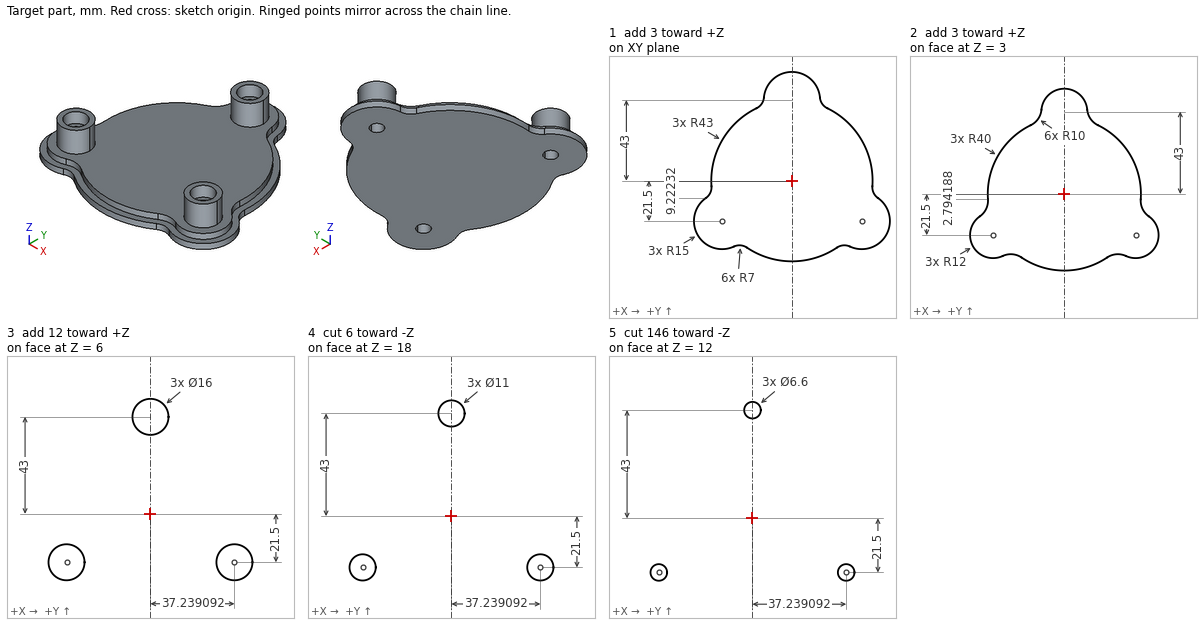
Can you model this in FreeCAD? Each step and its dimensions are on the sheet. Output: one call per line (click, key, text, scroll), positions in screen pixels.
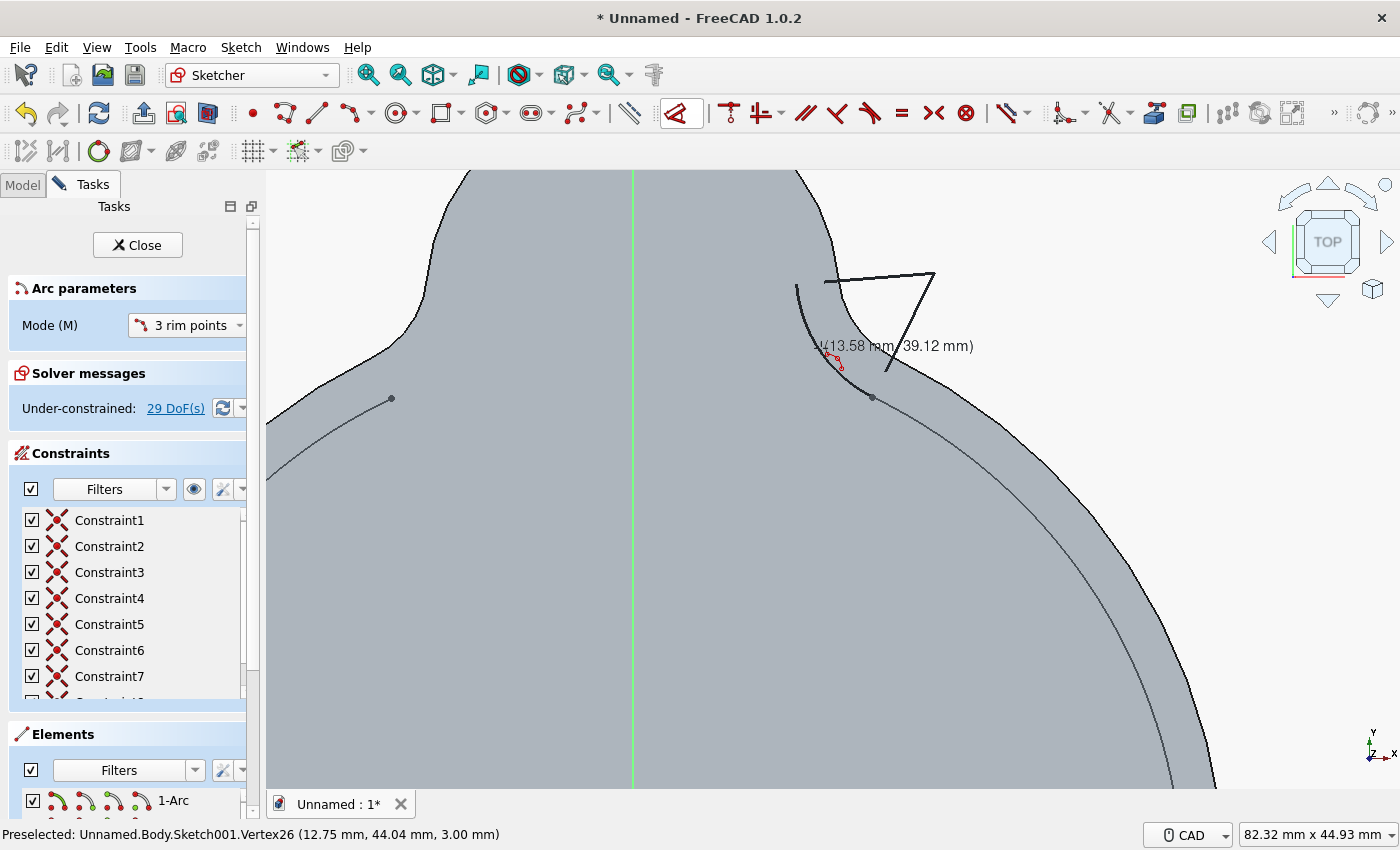
click(821, 349)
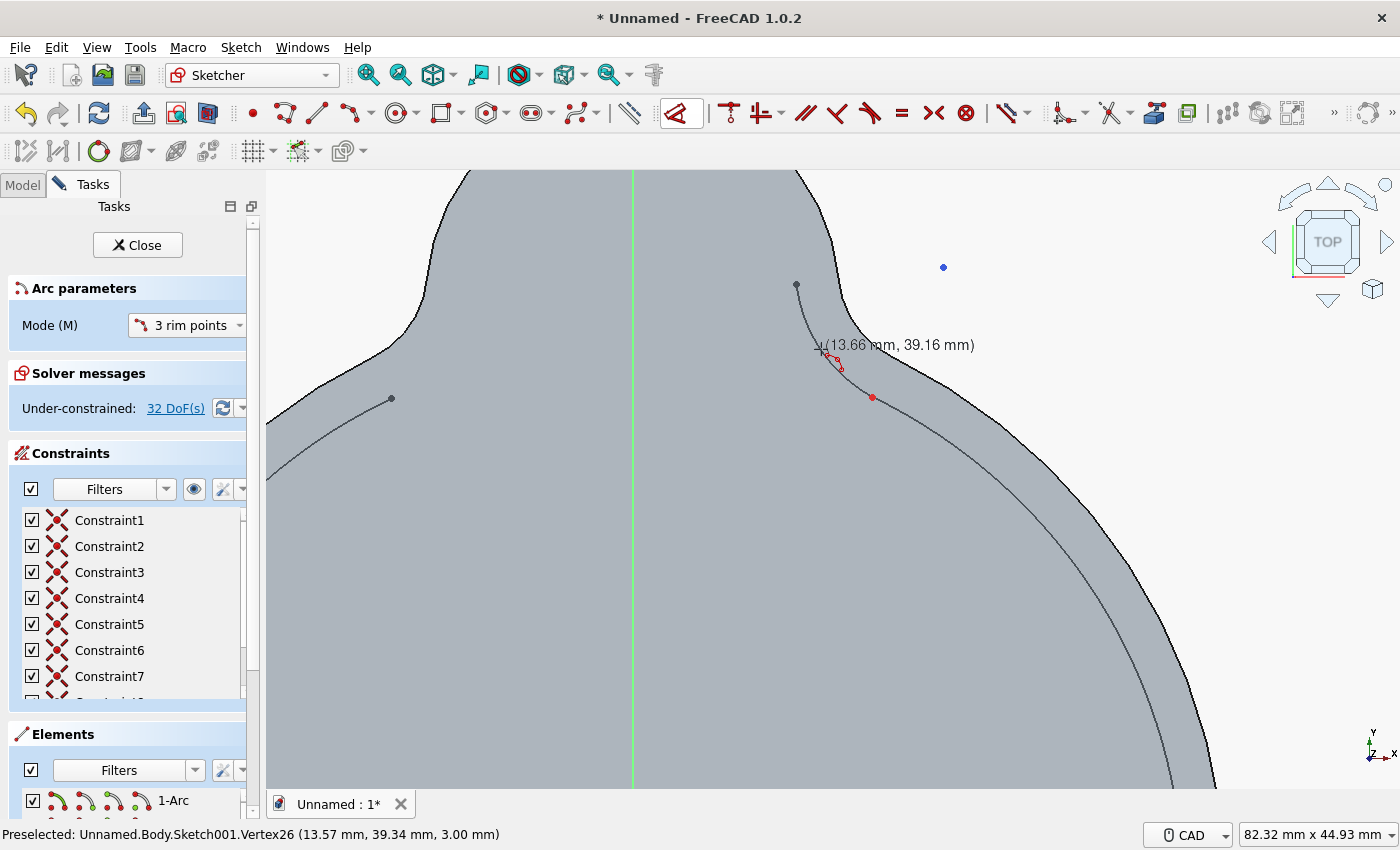
click(797, 284)
click(468, 283)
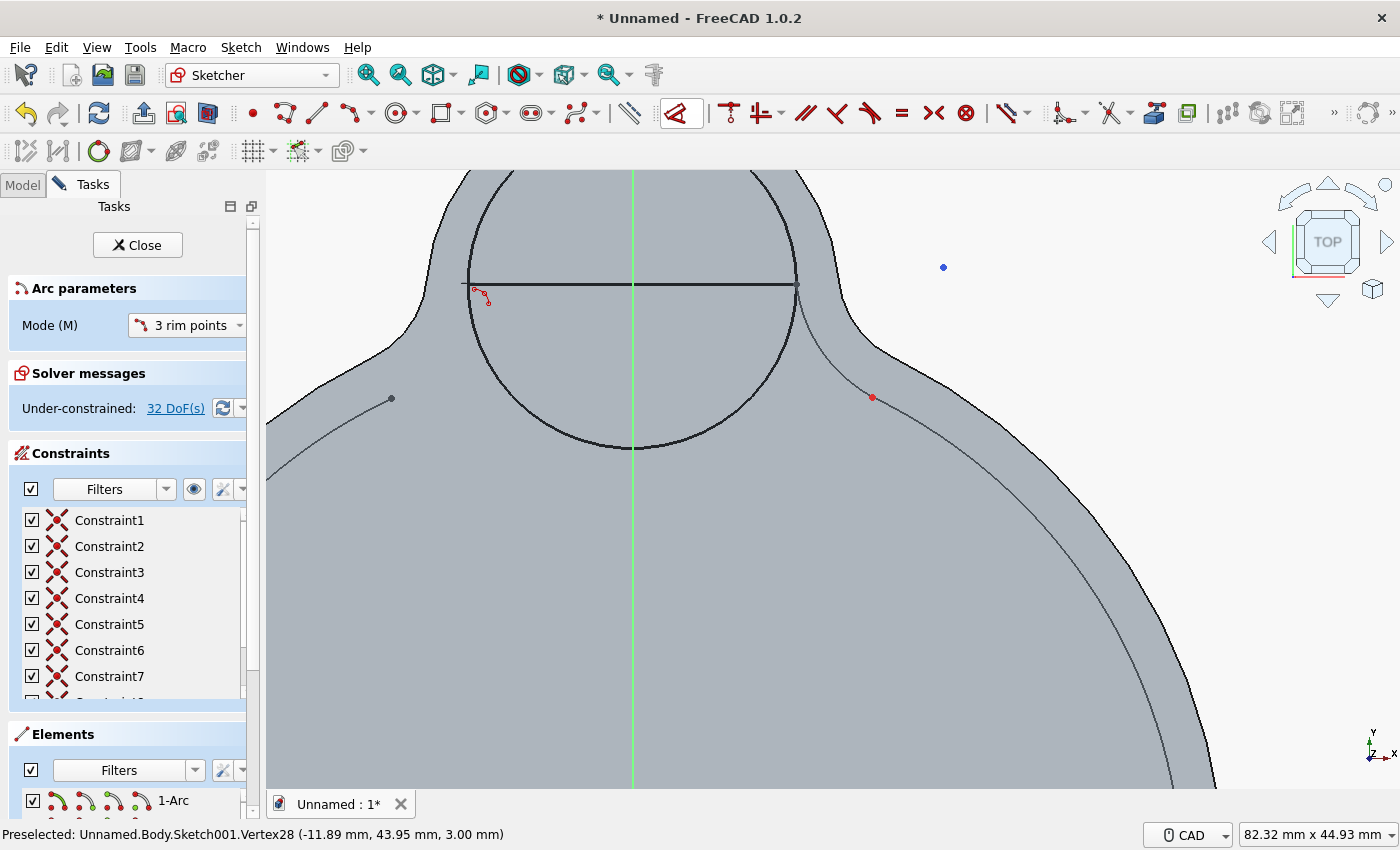
scroll(821, 347, down, 6)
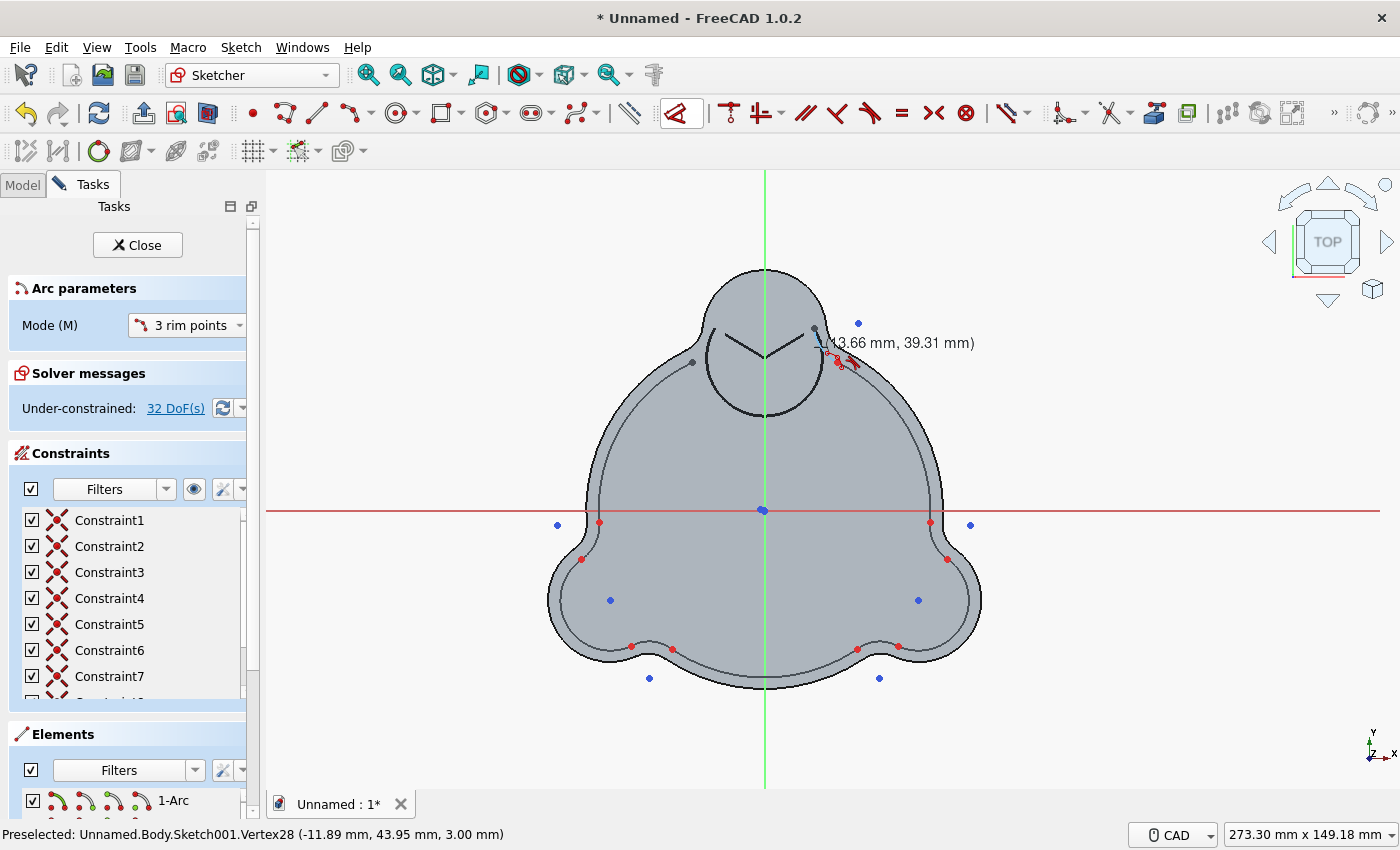
click(779, 285)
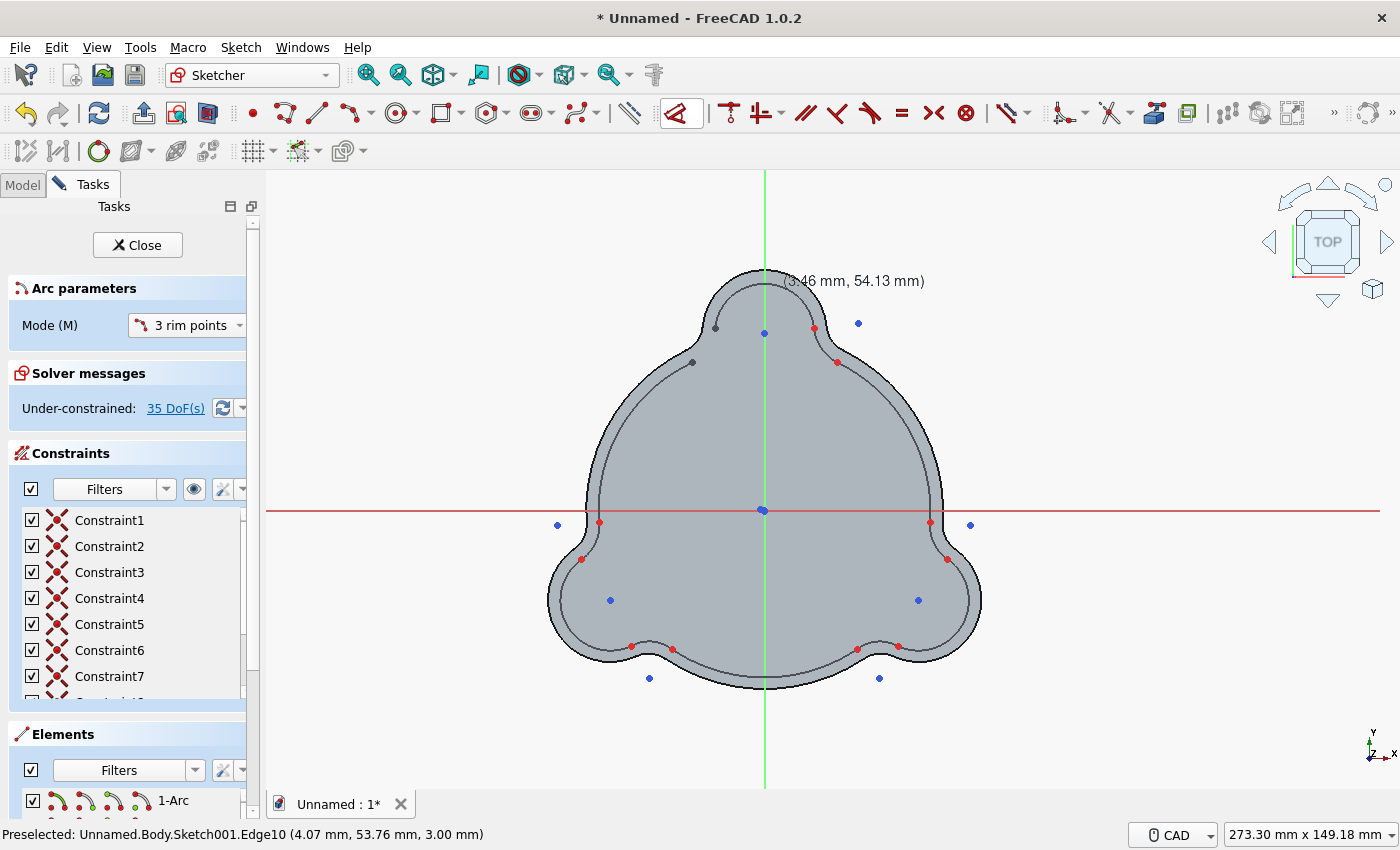
click(715, 328)
click(692, 363)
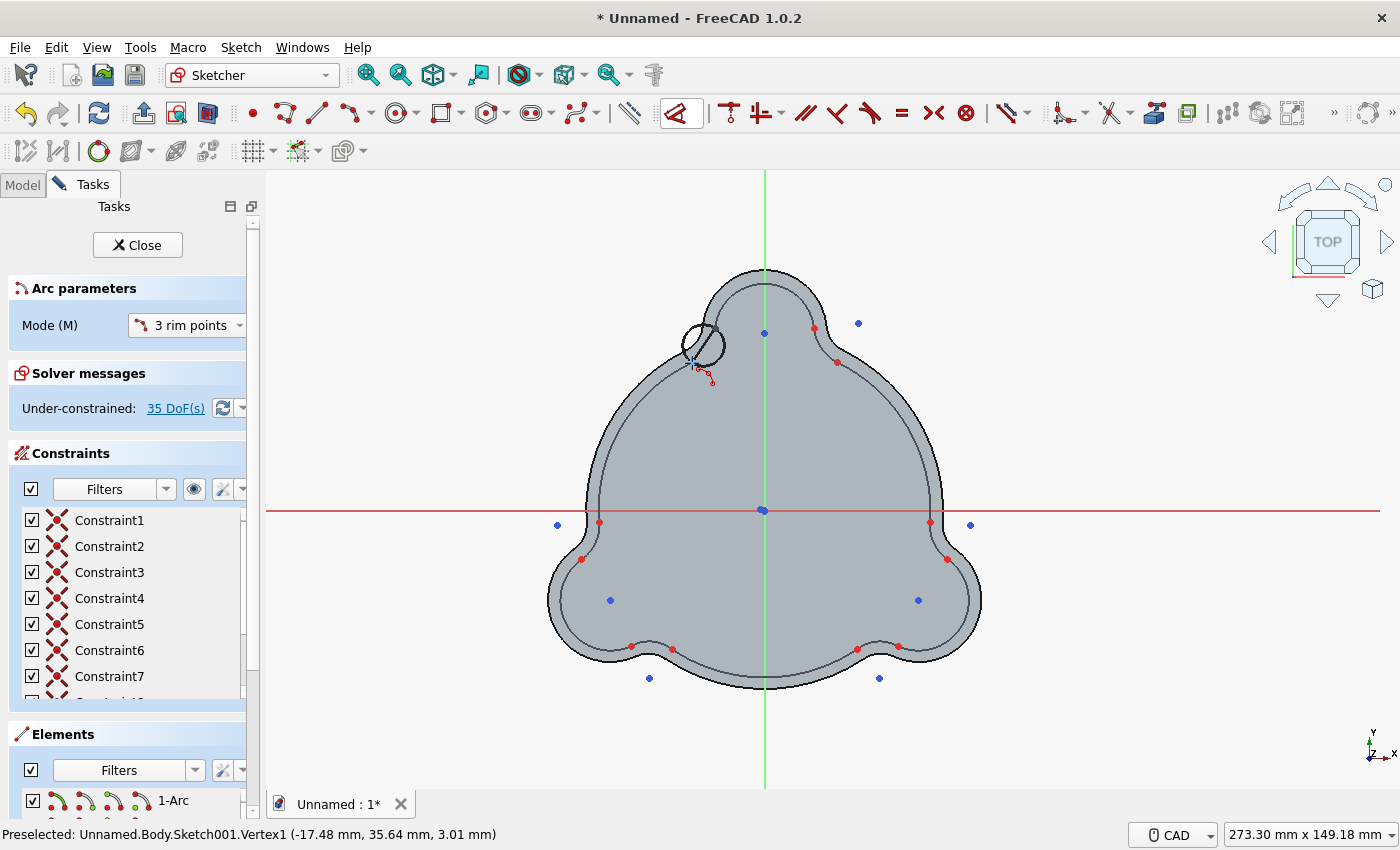
scroll(708, 348, up, 6)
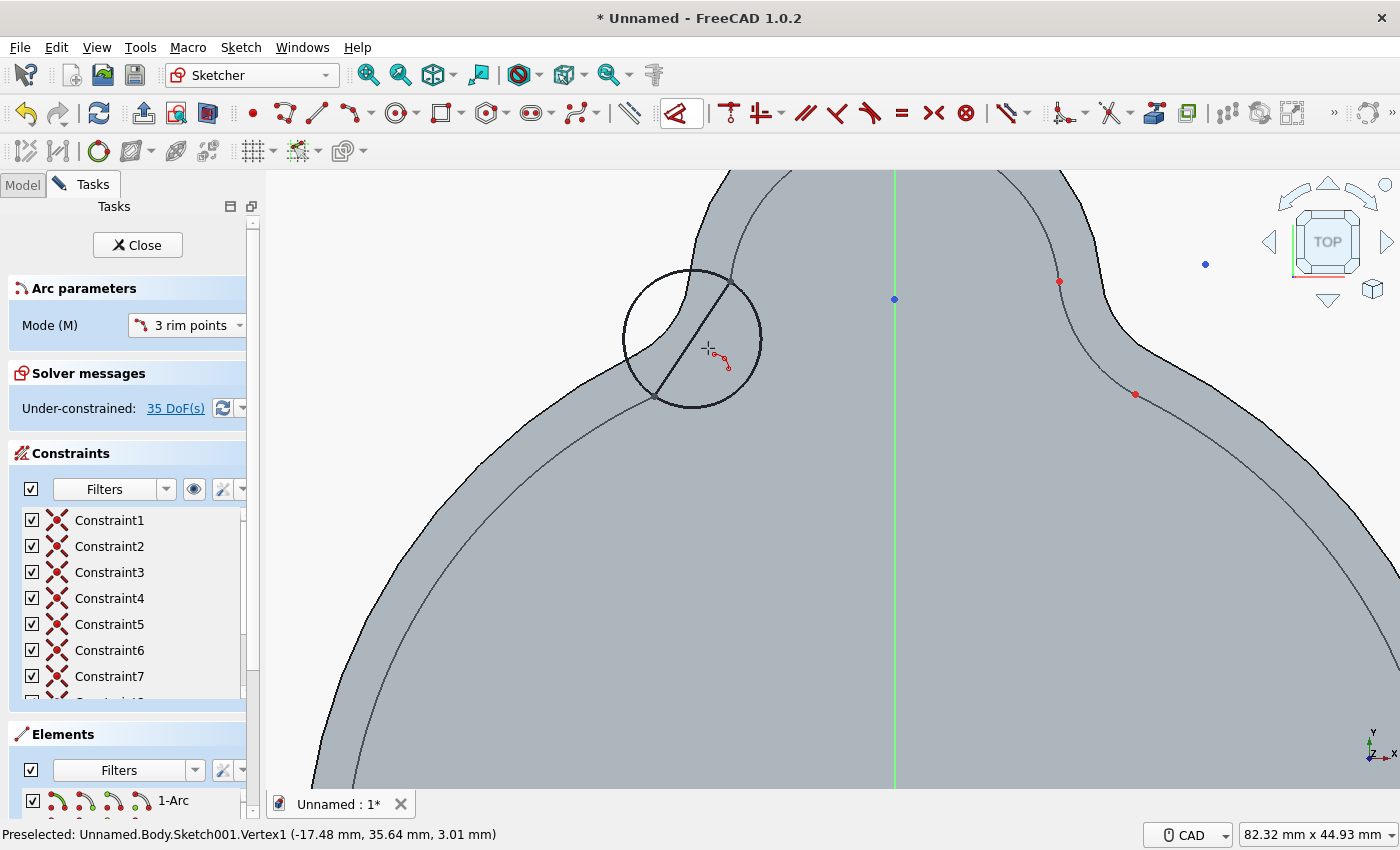
click(707, 346)
key(Escape)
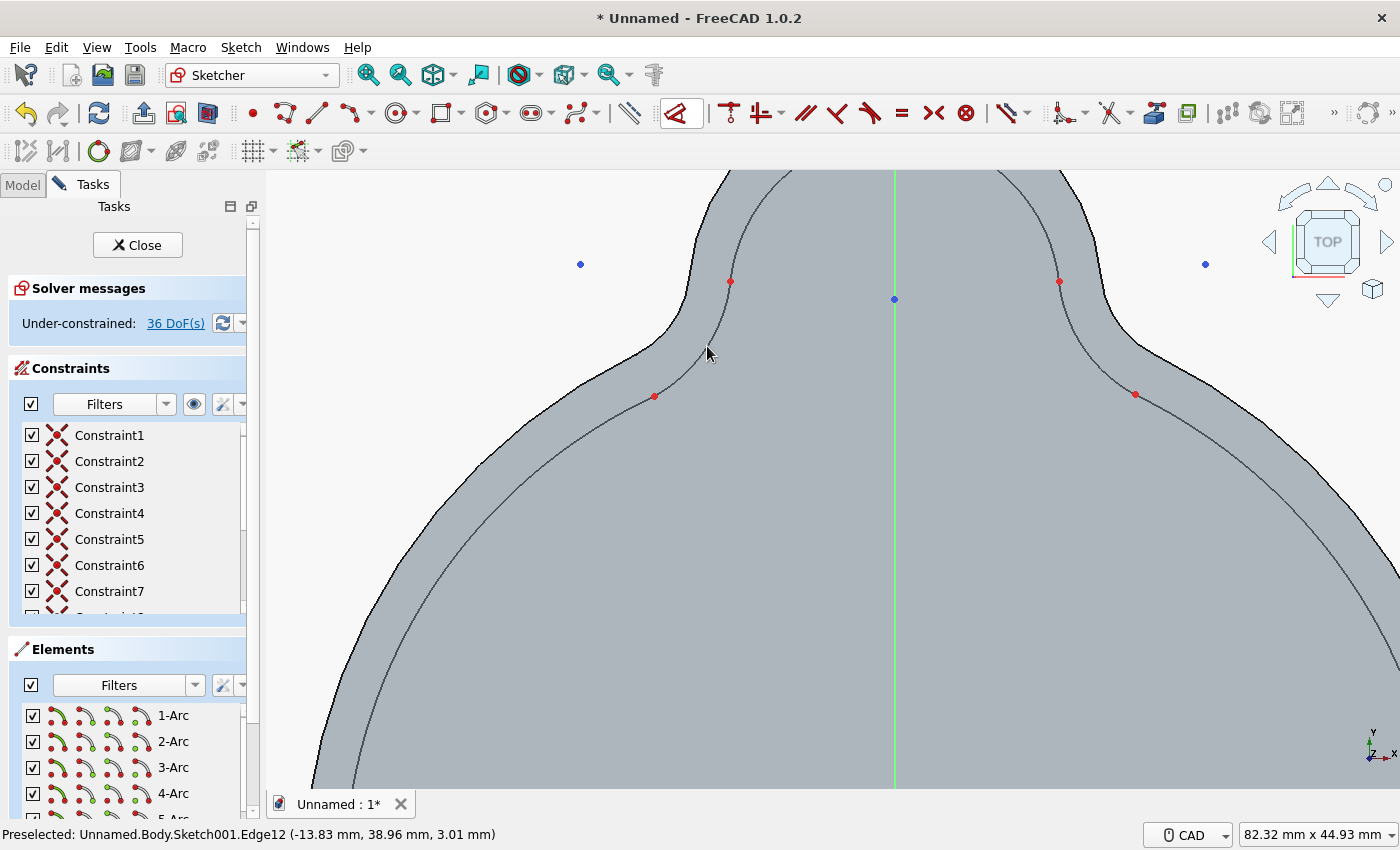
click(496, 509)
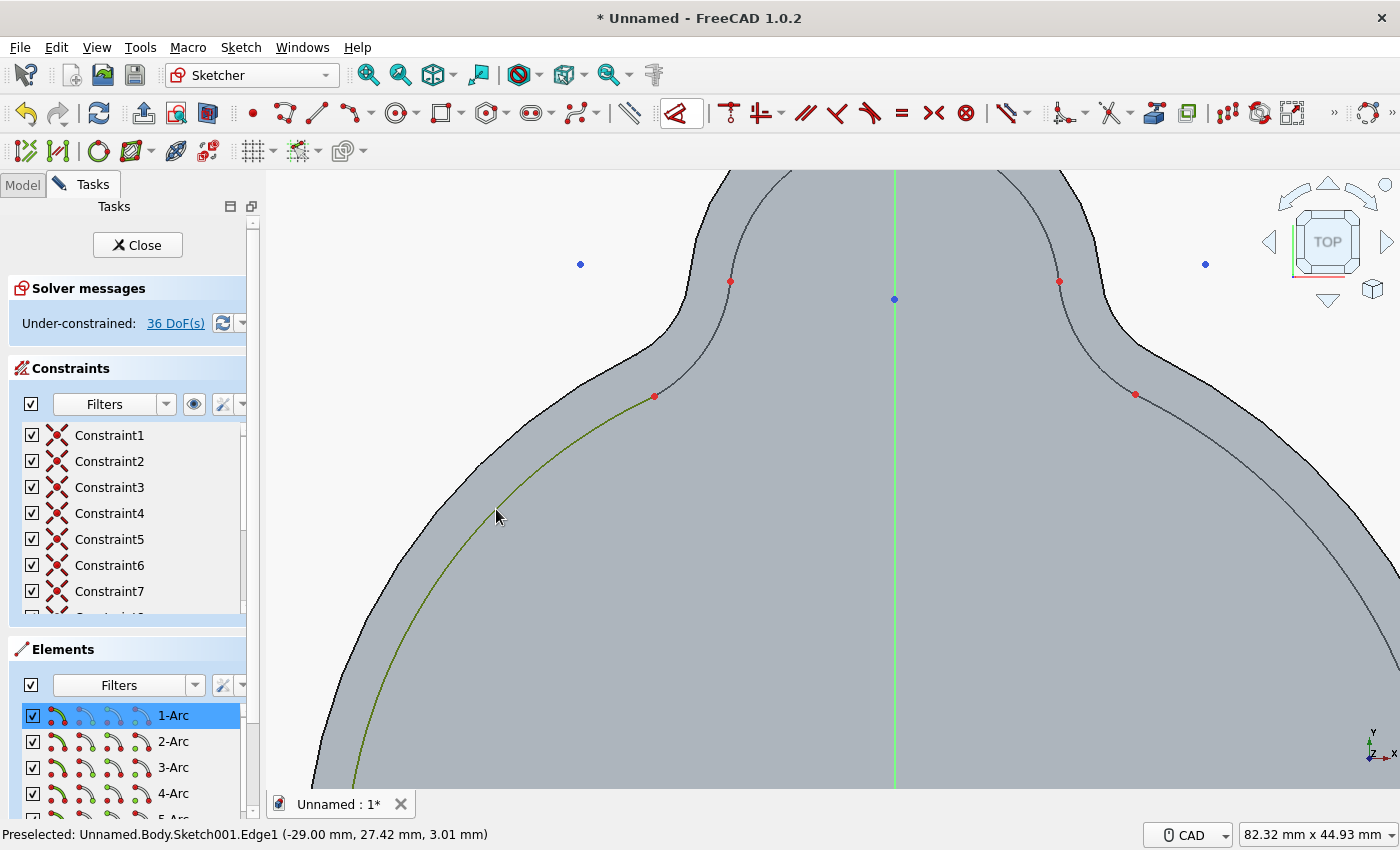
scroll(708, 348, down, 6)